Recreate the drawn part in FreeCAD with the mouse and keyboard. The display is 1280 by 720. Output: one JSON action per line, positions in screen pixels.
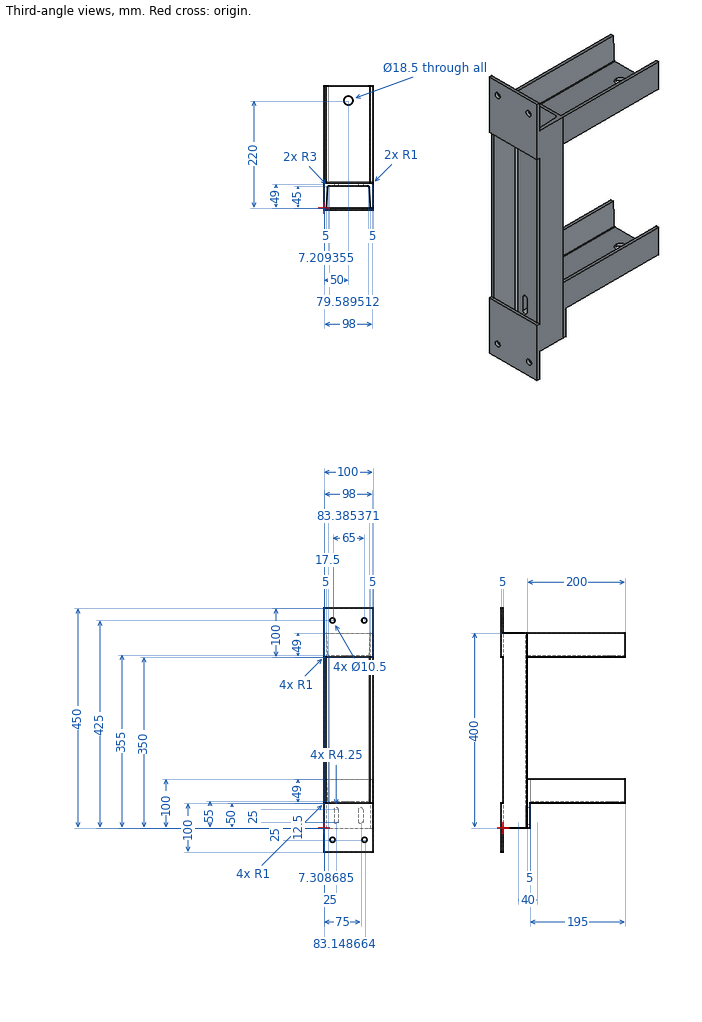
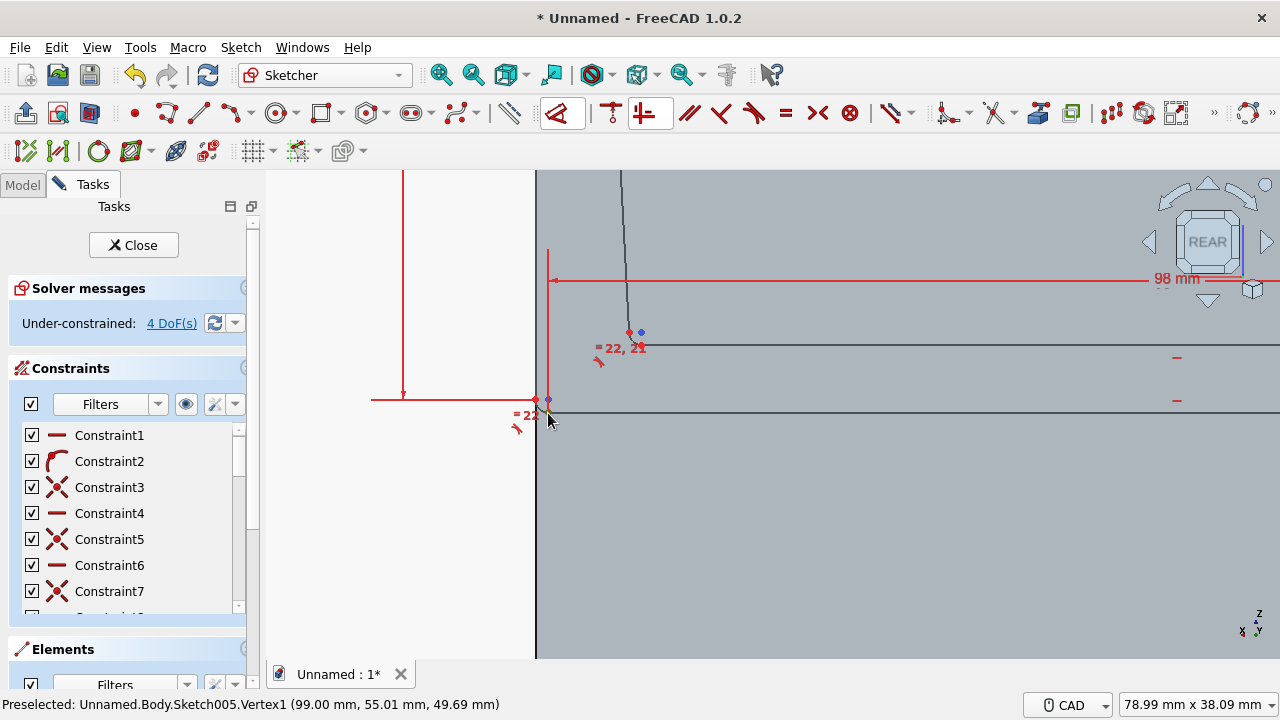
{"action": "left_click", "coordinate": [580, 114]}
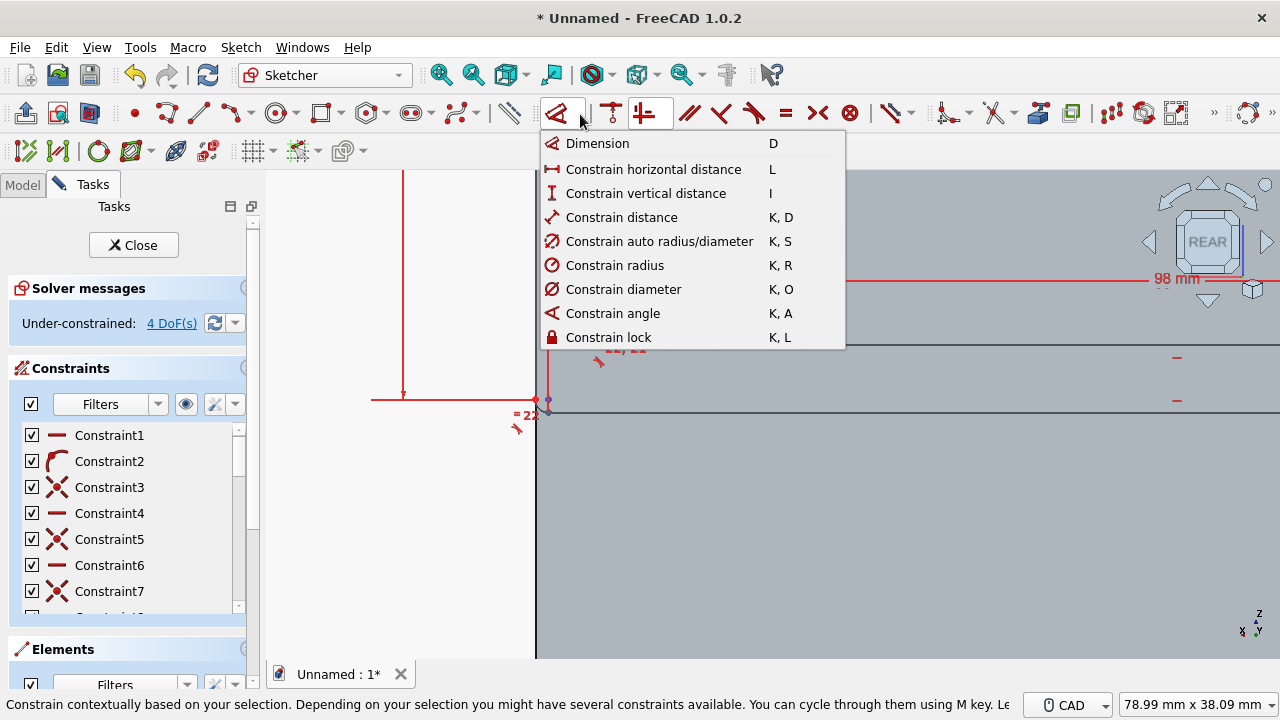
{"action": "left_click", "coordinate": [693, 193]}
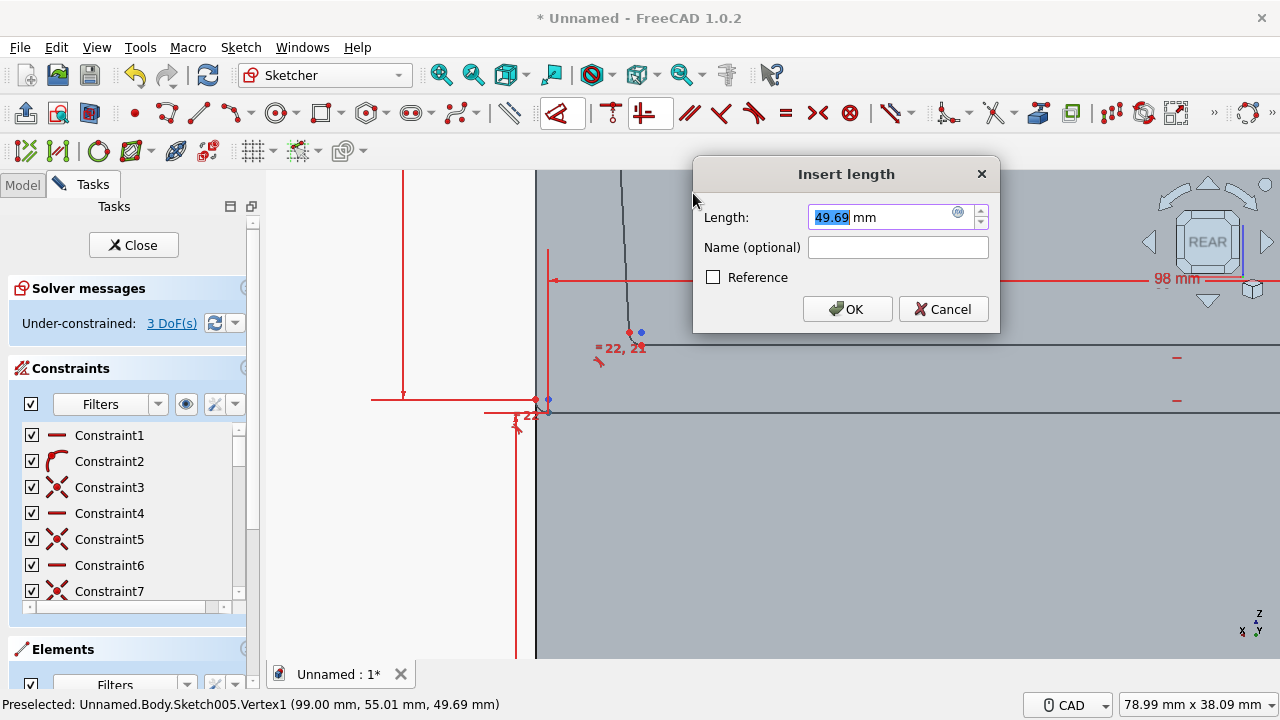
{"action": "type", "text": "50"}
{"action": "key", "text": "Return"}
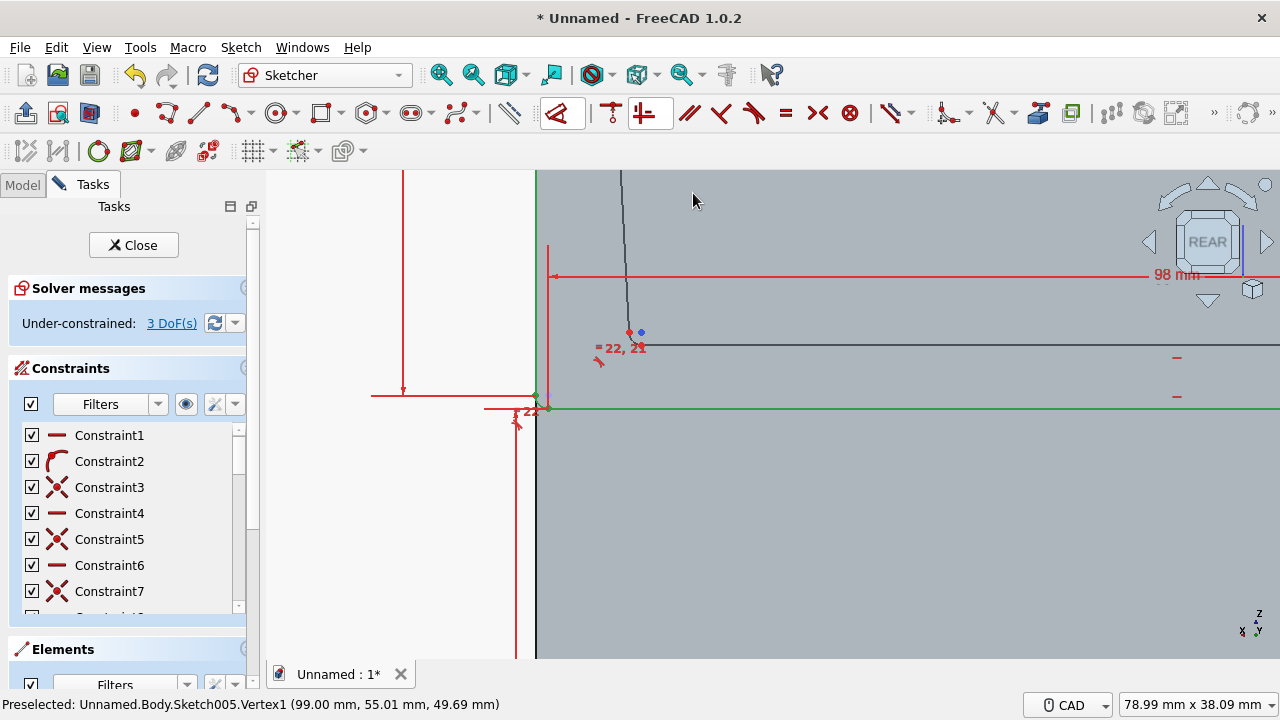
{"action": "scroll", "coordinate": [550, 416], "scroll_direction": "down", "scroll_amount": 7}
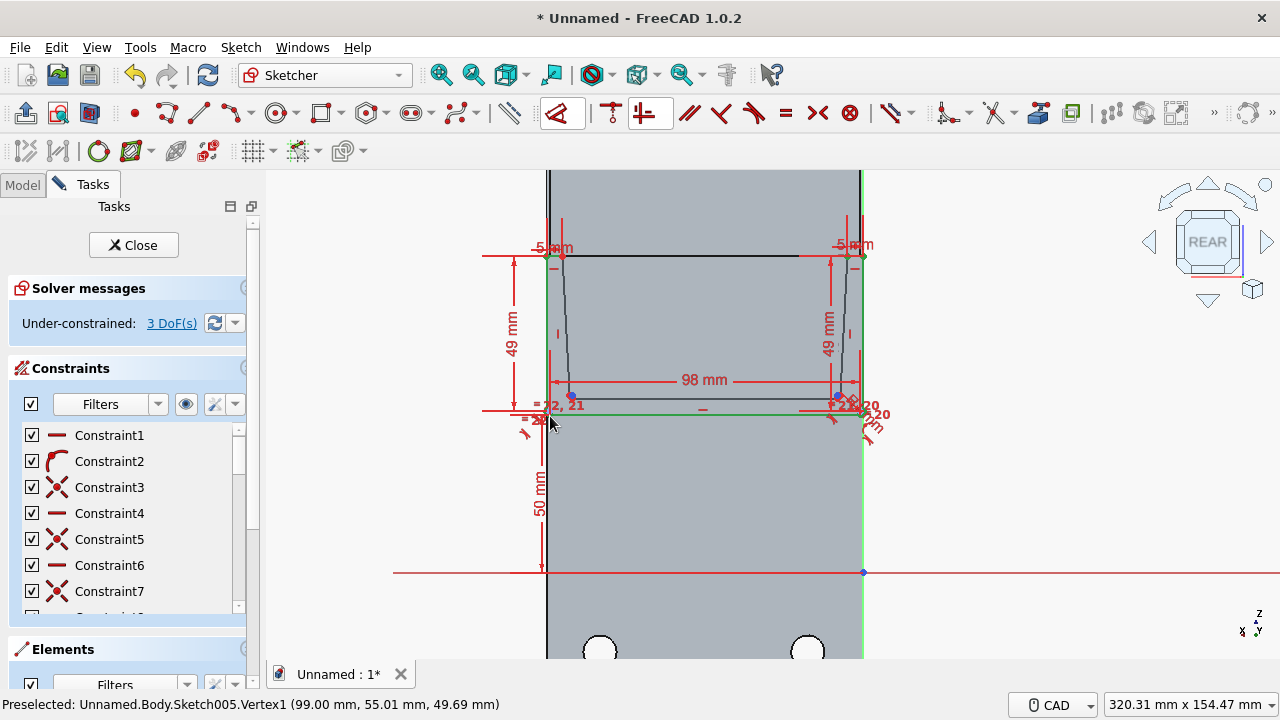
{"action": "scroll", "coordinate": [837, 399], "scroll_direction": "up", "scroll_amount": 7}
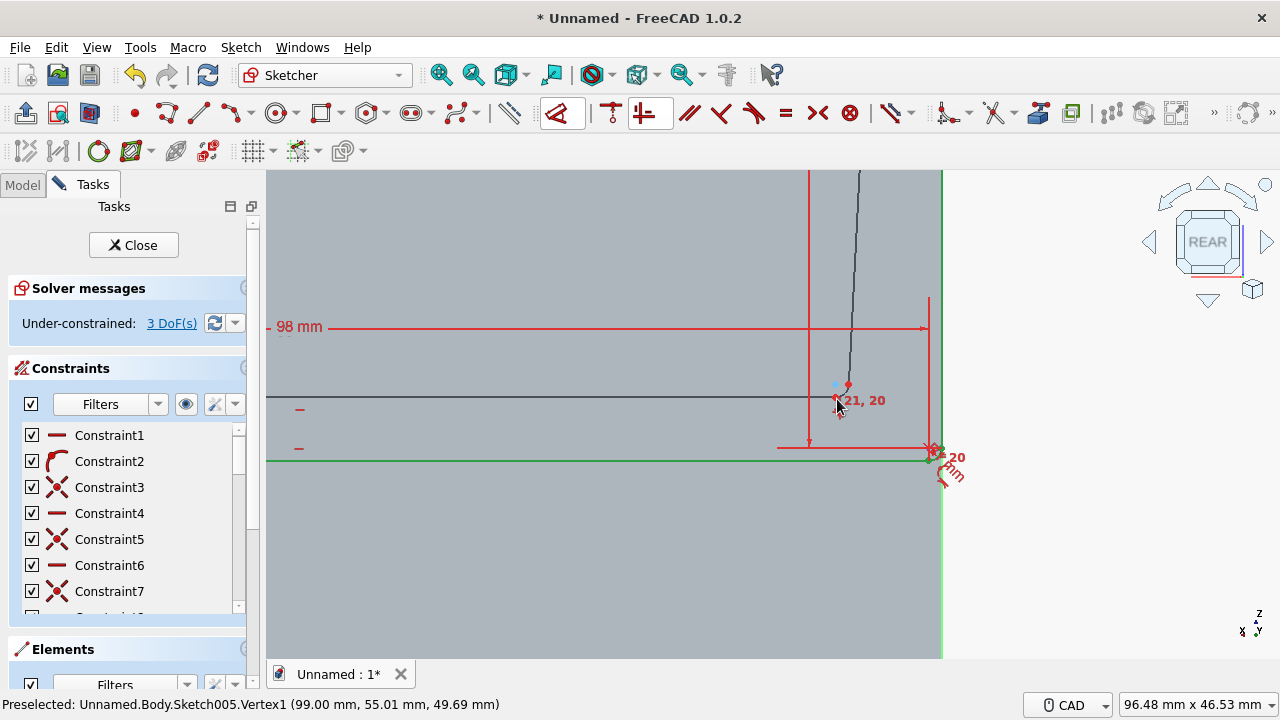
{"action": "left_click", "coordinate": [836, 397]}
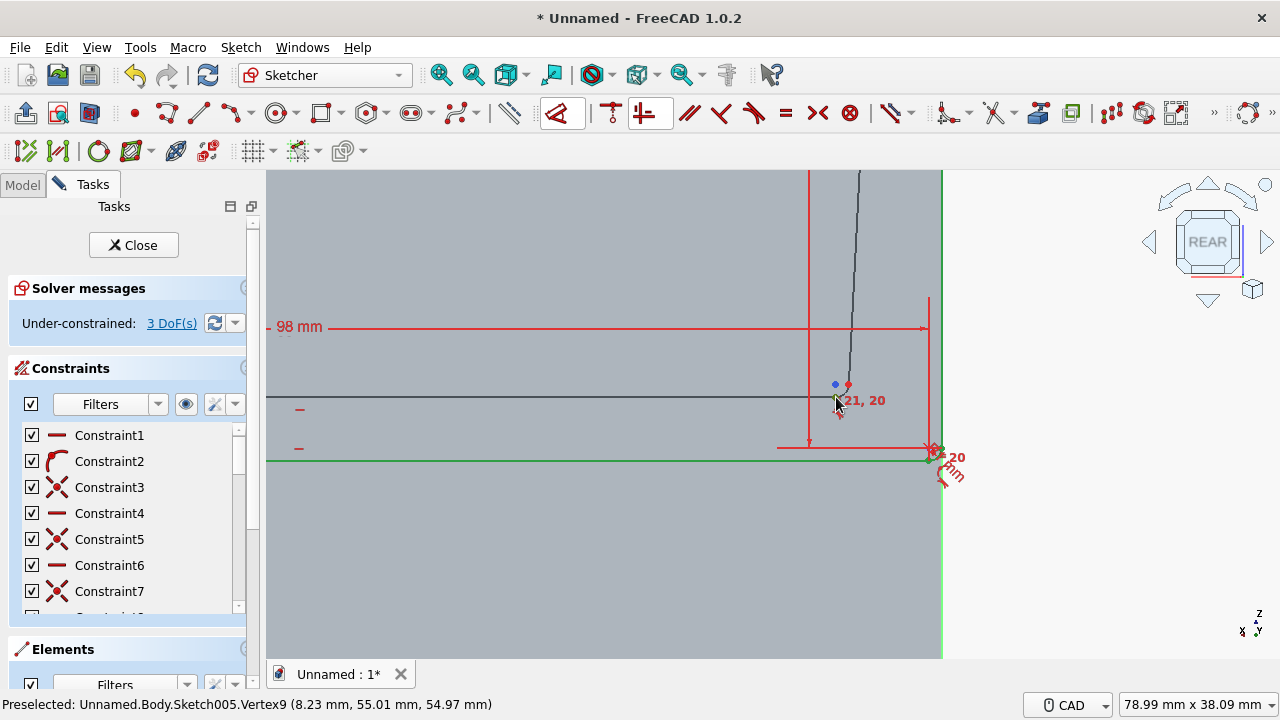
{"action": "key", "text": "i"}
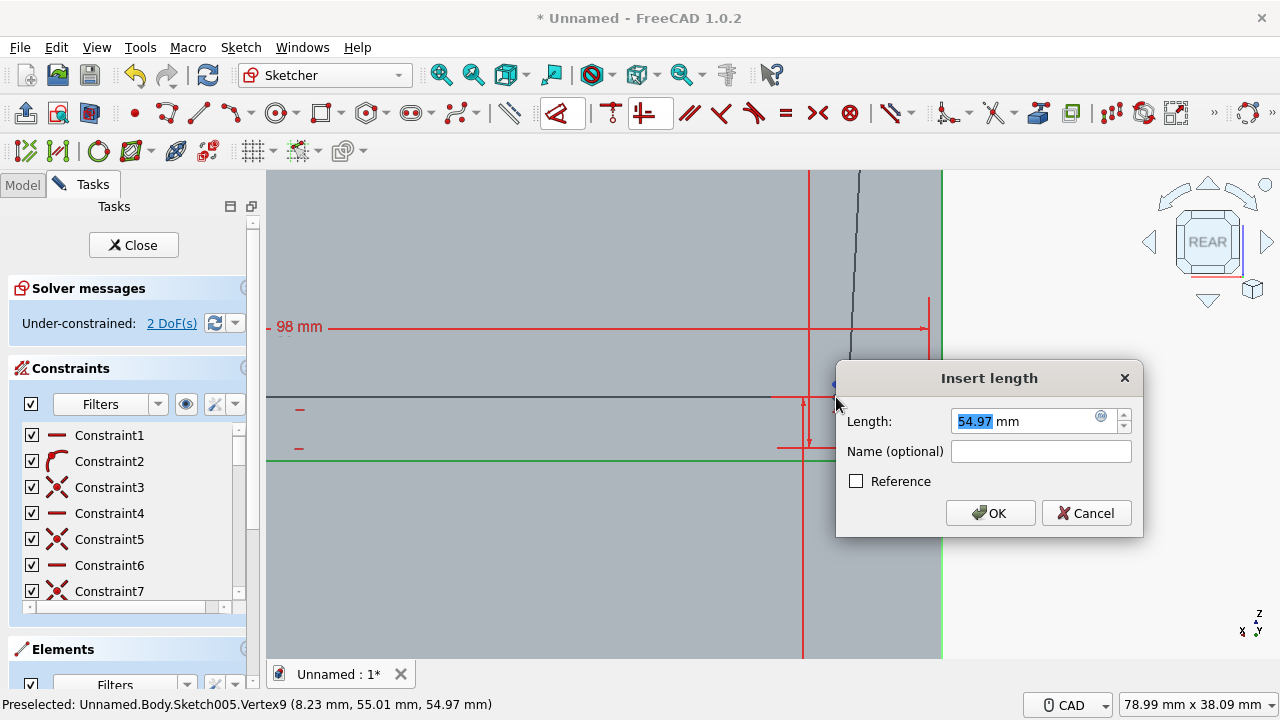
{"action": "type", "text": "55"}
{"action": "key", "text": "Return"}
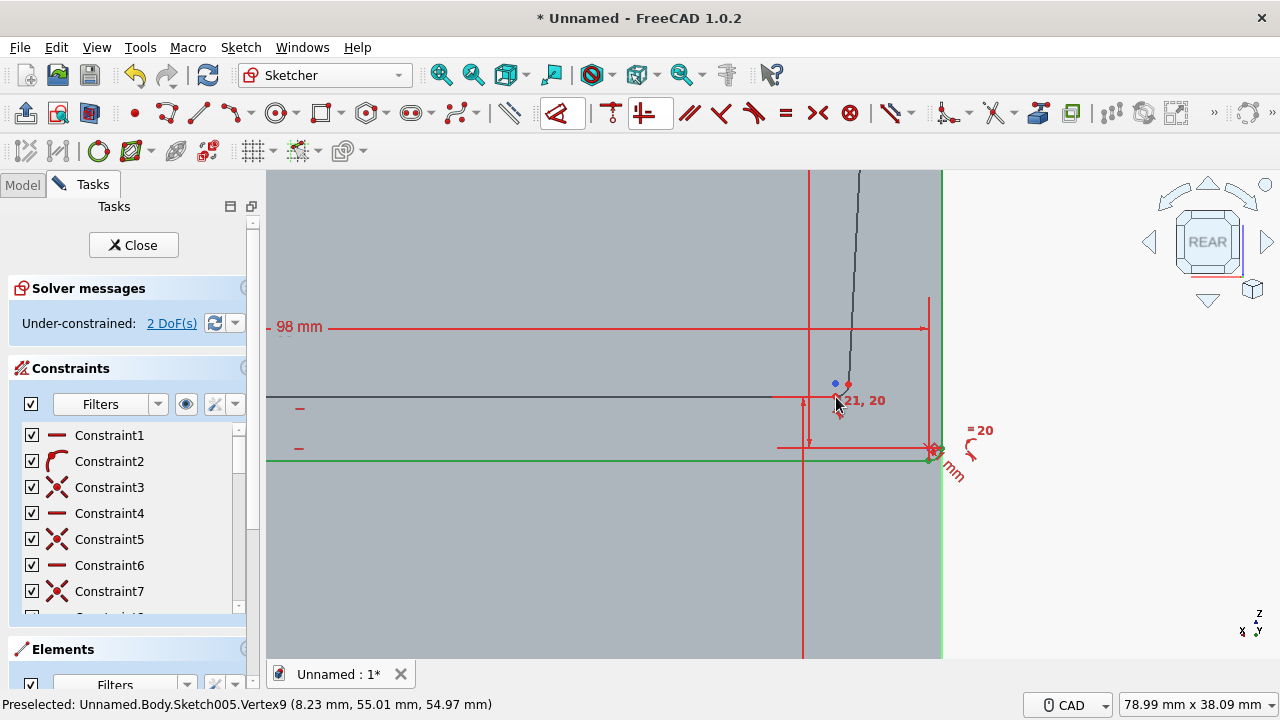
{"action": "scroll", "coordinate": [837, 399], "scroll_direction": "down", "scroll_amount": 7}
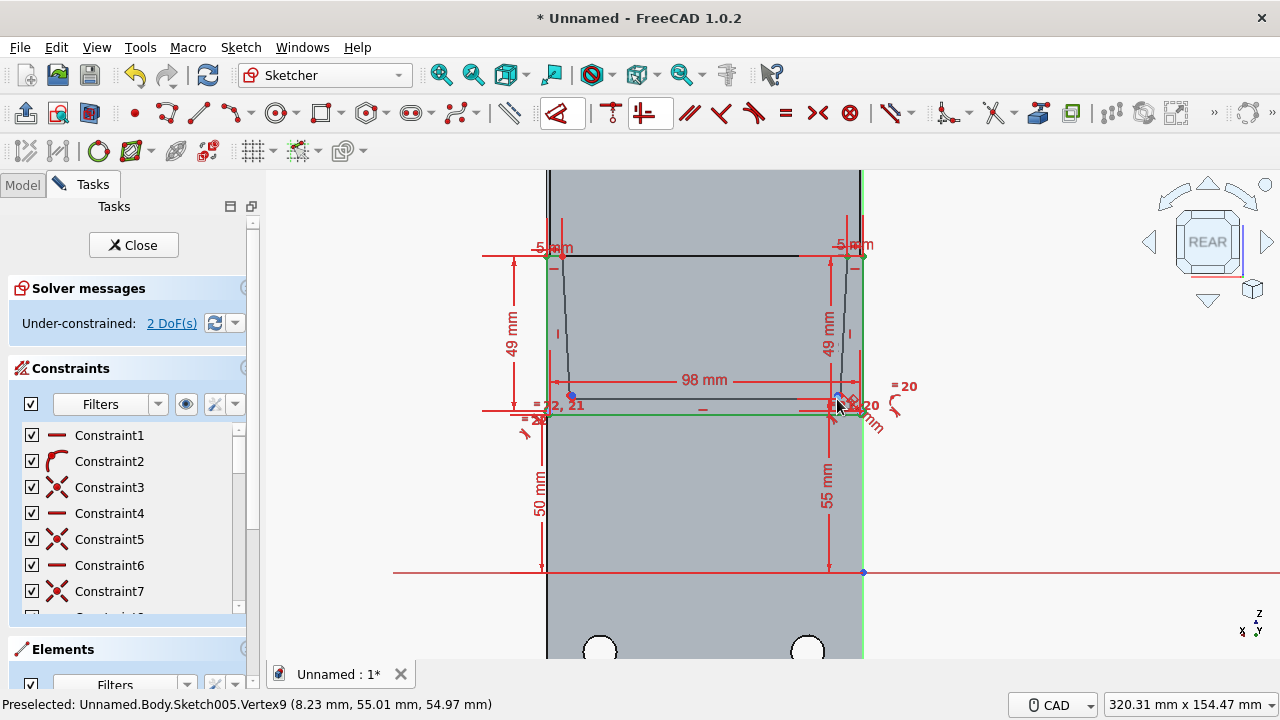
{"action": "left_click", "coordinate": [758, 399]}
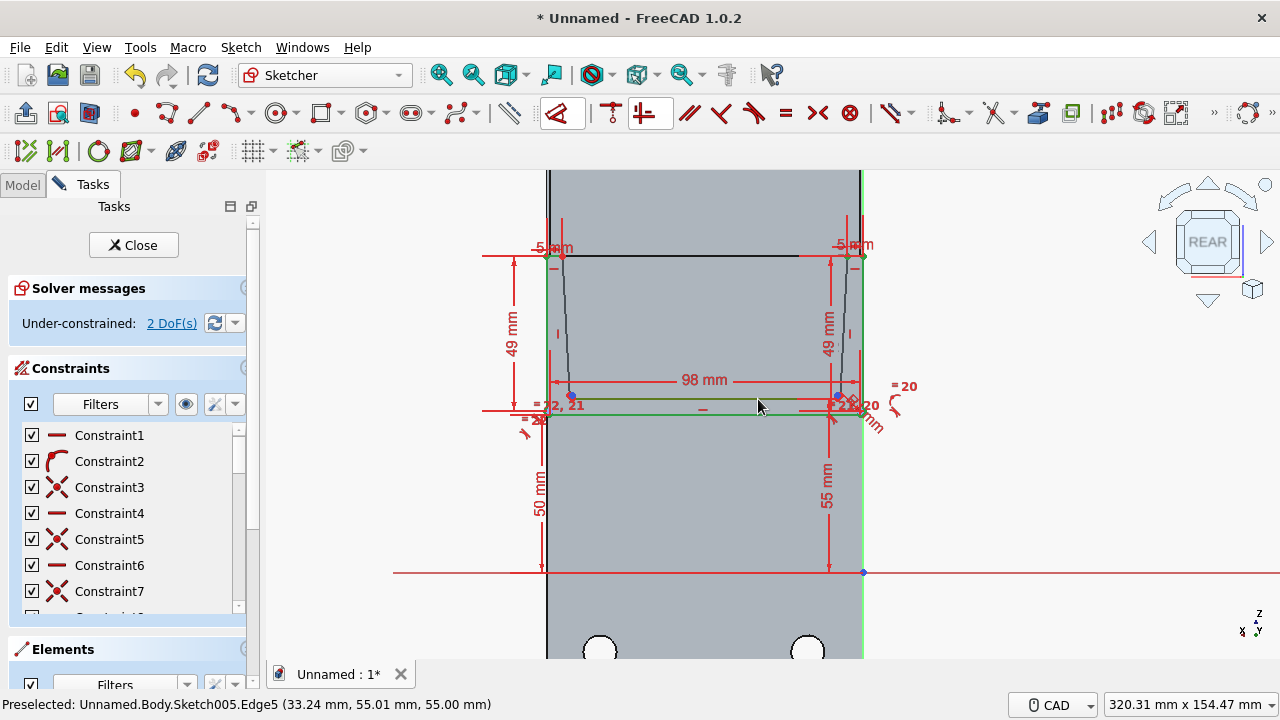
{"action": "key", "text": "l"}